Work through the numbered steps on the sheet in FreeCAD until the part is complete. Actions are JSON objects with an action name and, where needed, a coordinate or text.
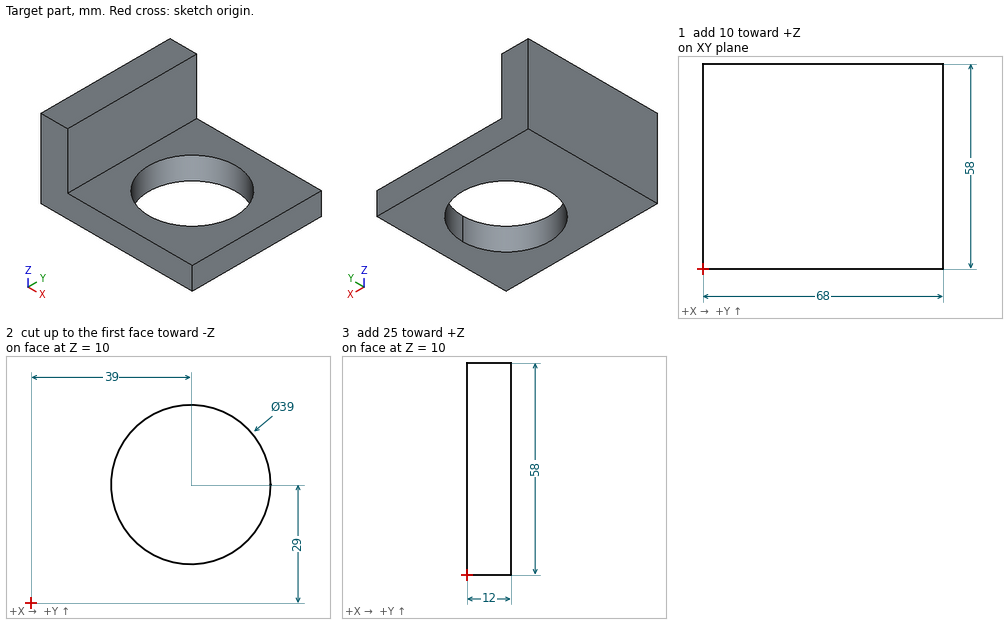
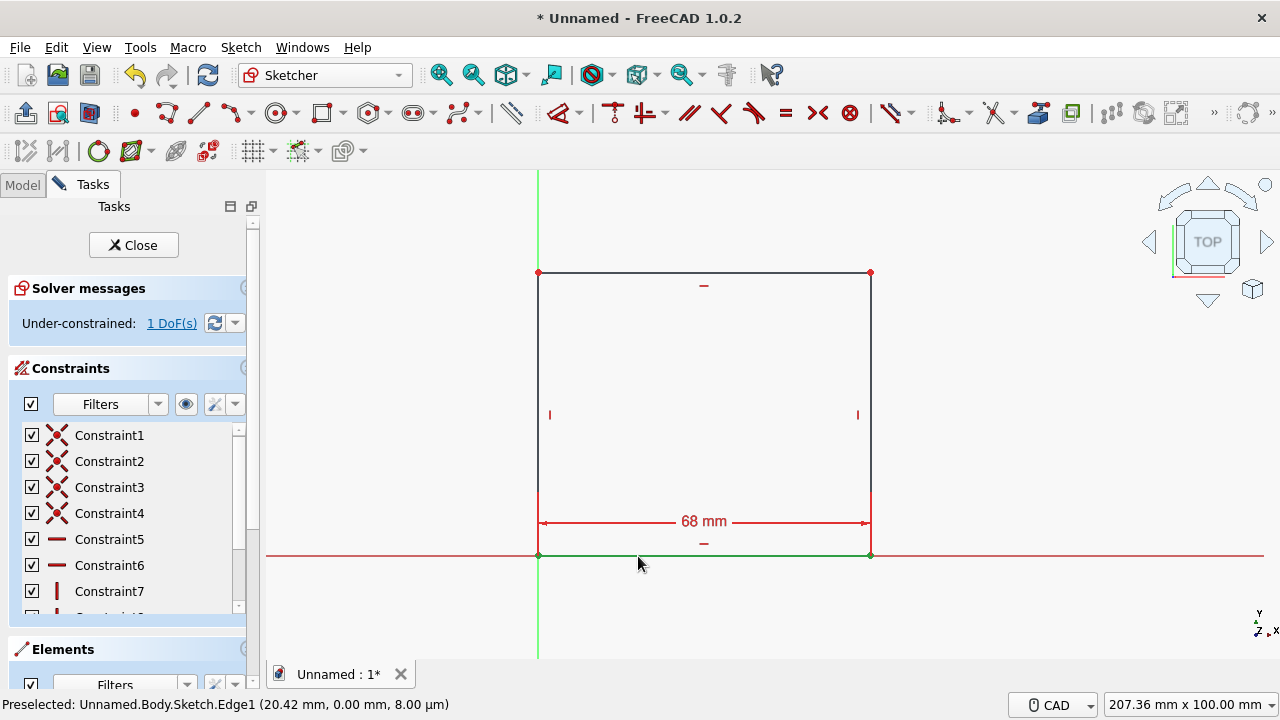
{"action": "left_click", "coordinate": [871, 471]}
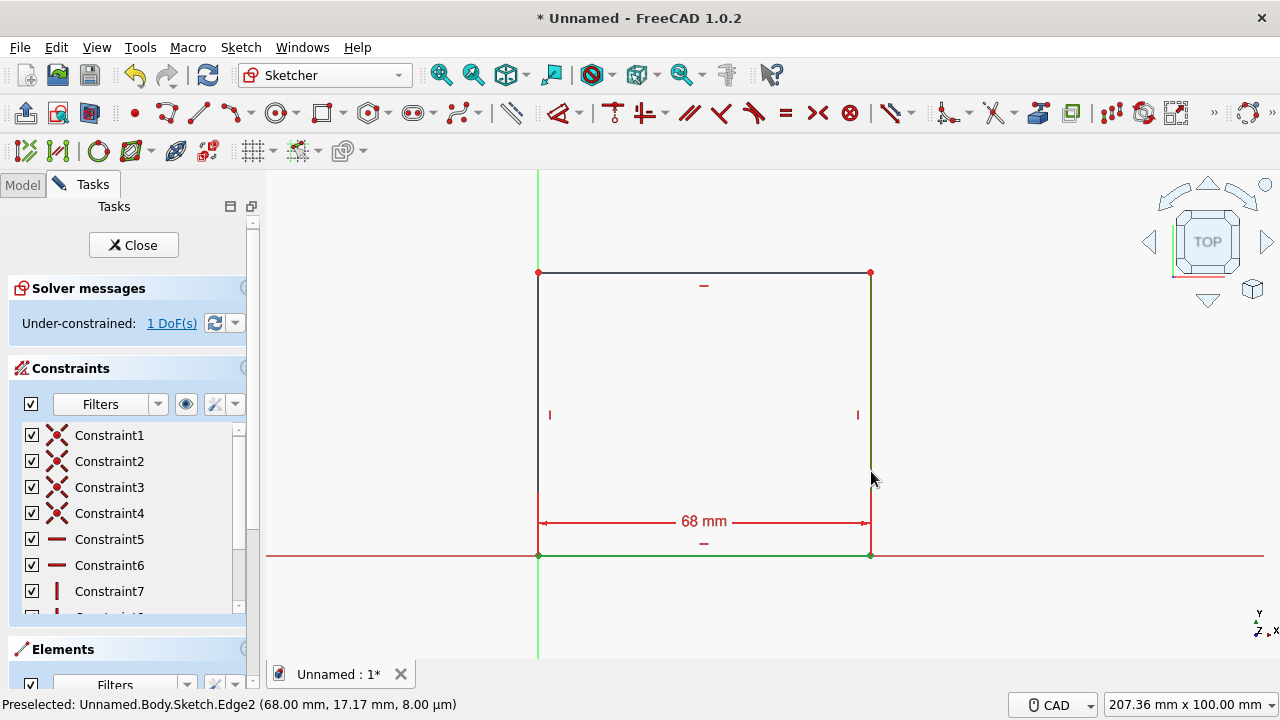
{"action": "left_click", "coordinate": [582, 114]}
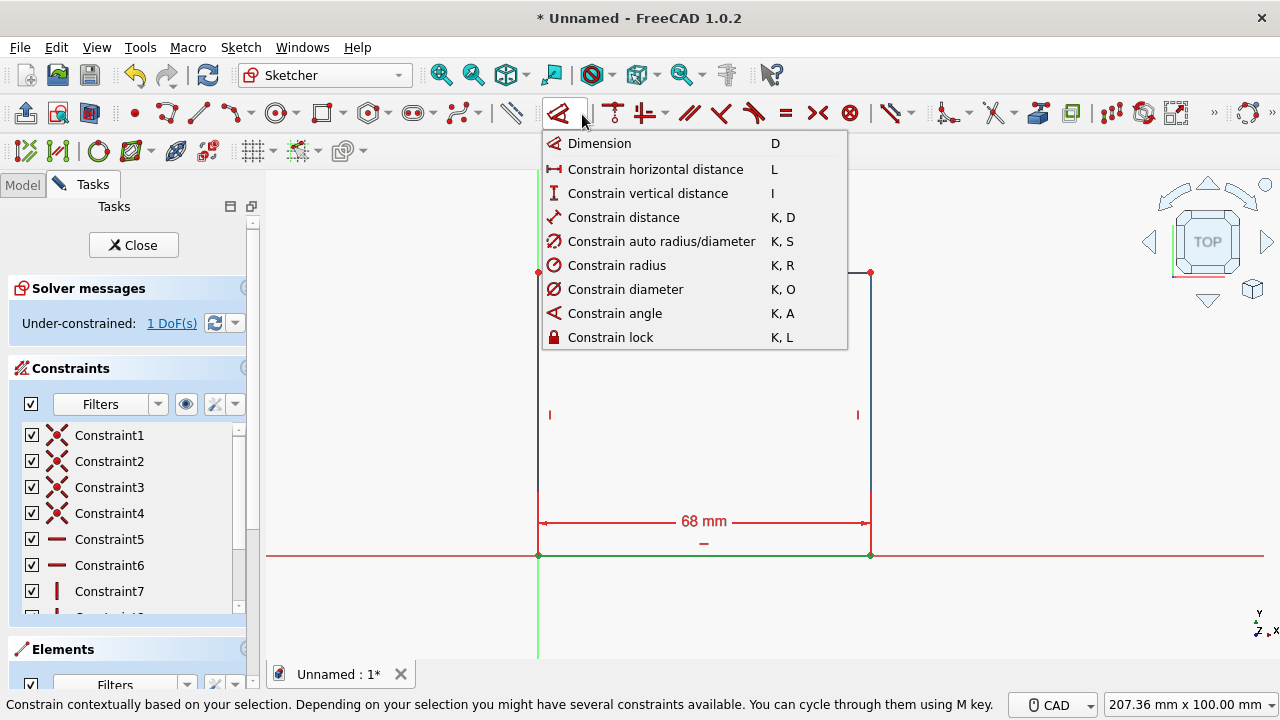
{"action": "left_click", "coordinate": [695, 193]}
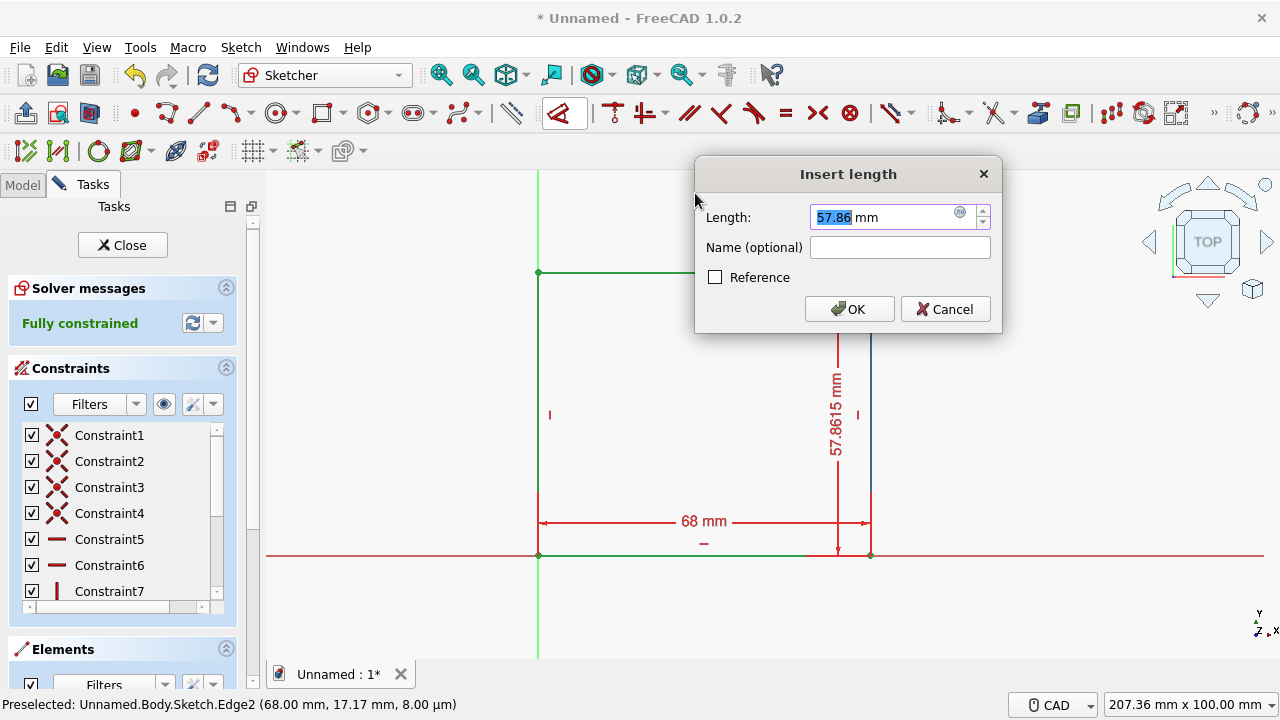
{"action": "type", "text": "58"}
{"action": "key", "text": "Return"}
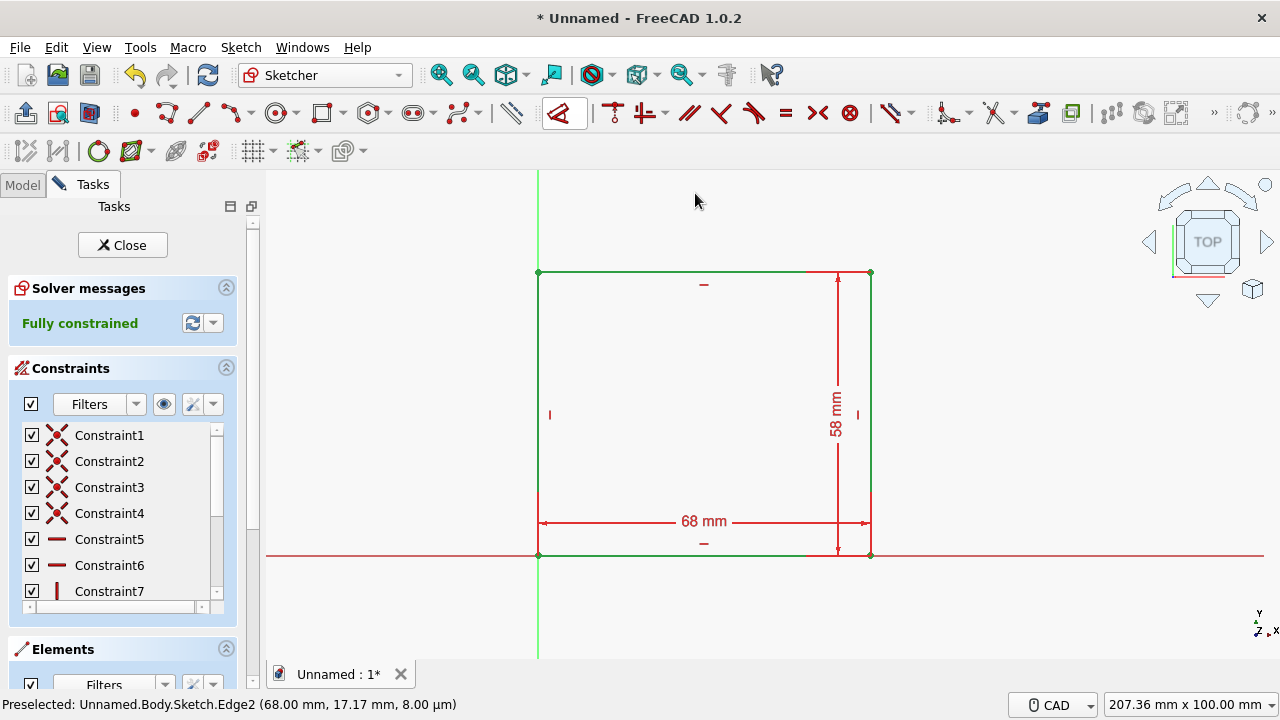
{"action": "left_click", "coordinate": [123, 245]}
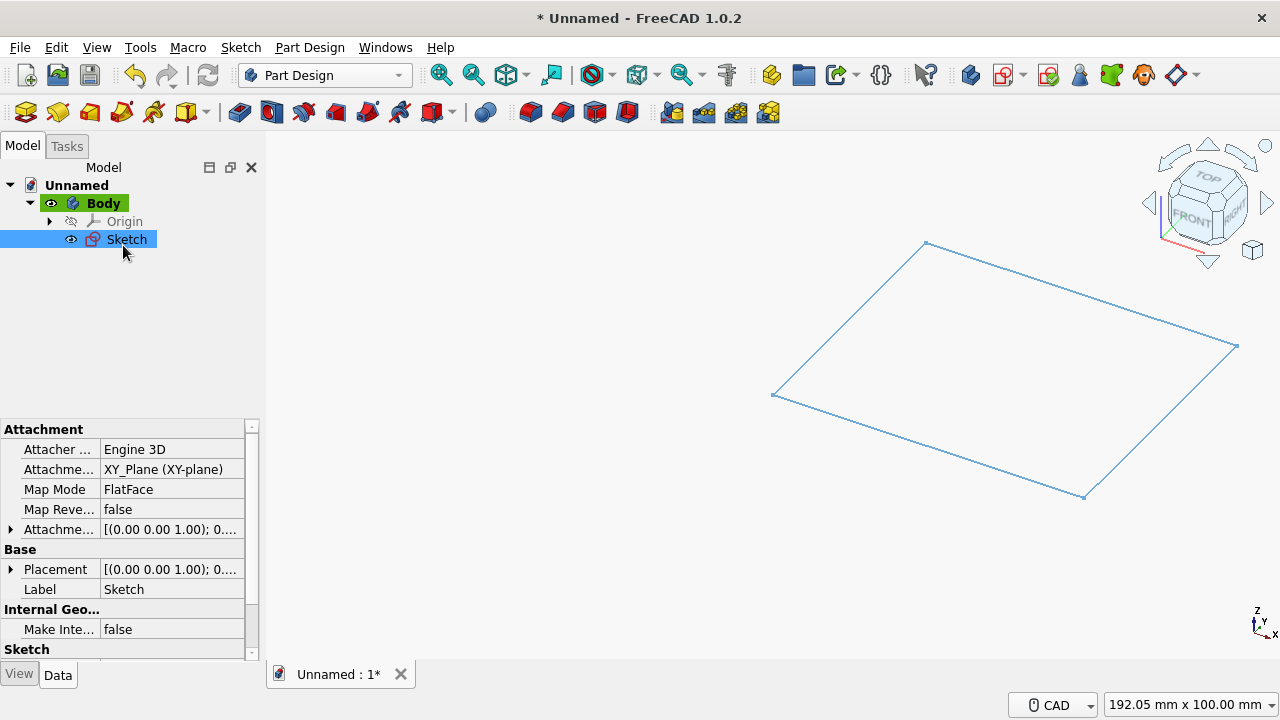
{"action": "left_click", "coordinate": [26, 112]}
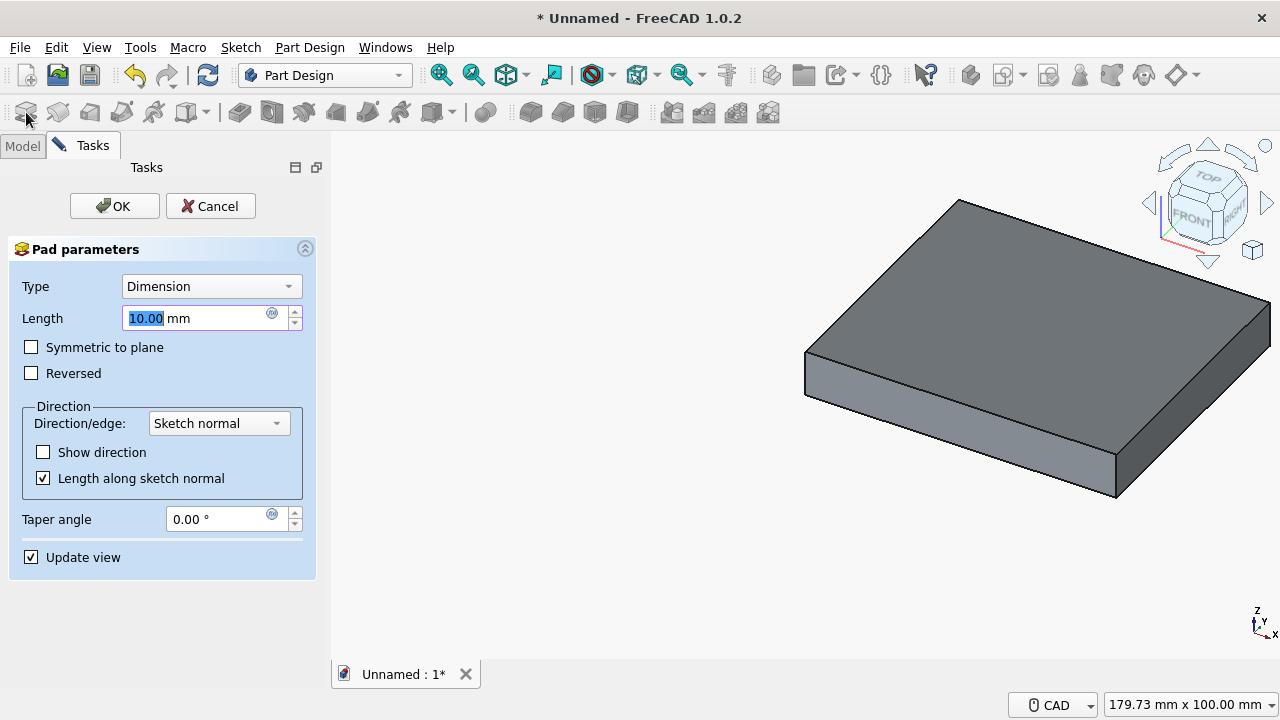
{"action": "type", "text": "10"}
{"action": "key", "text": "Tab"}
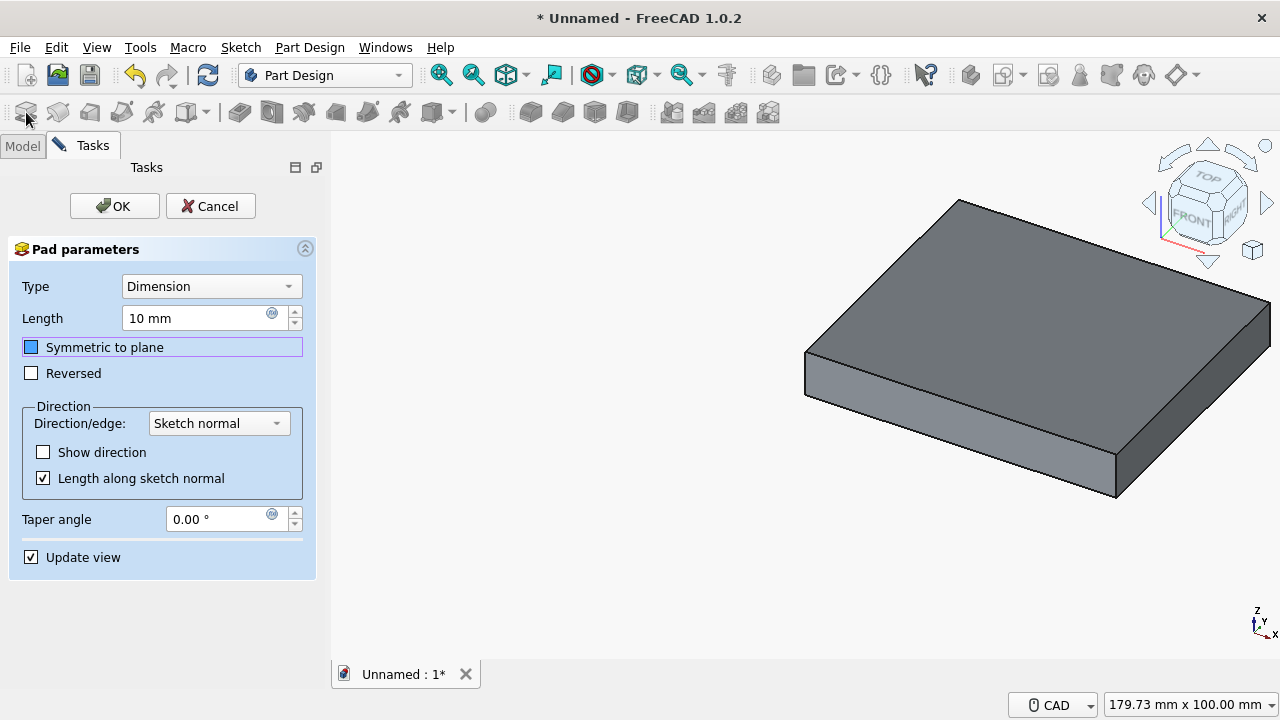
{"action": "left_click", "coordinate": [115, 206]}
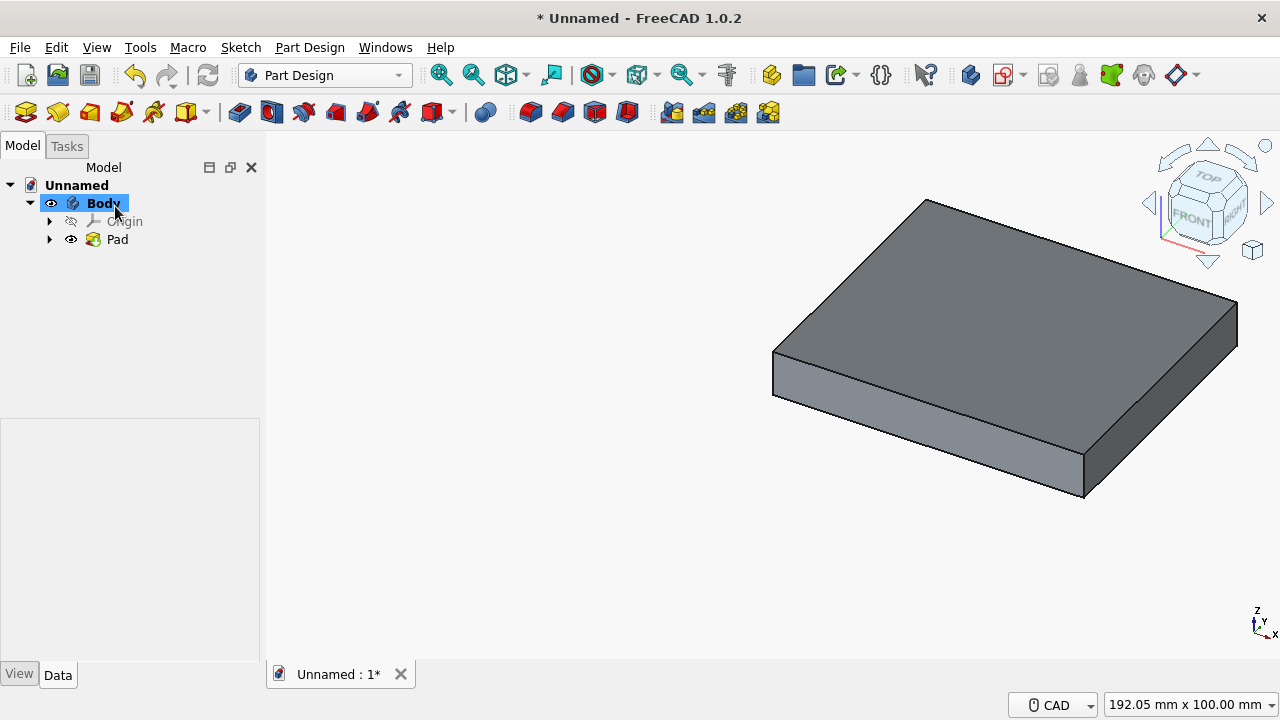
{"action": "left_click", "coordinate": [1005, 326]}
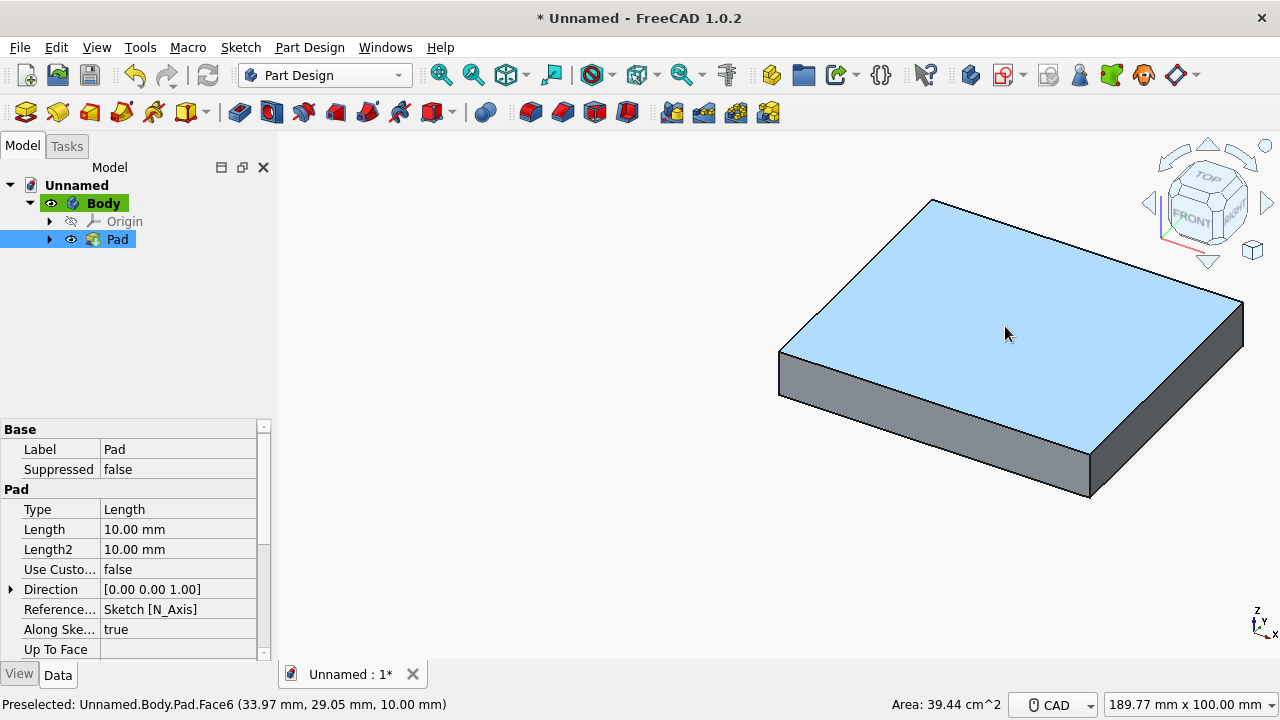
{"action": "left_click", "coordinate": [1004, 76]}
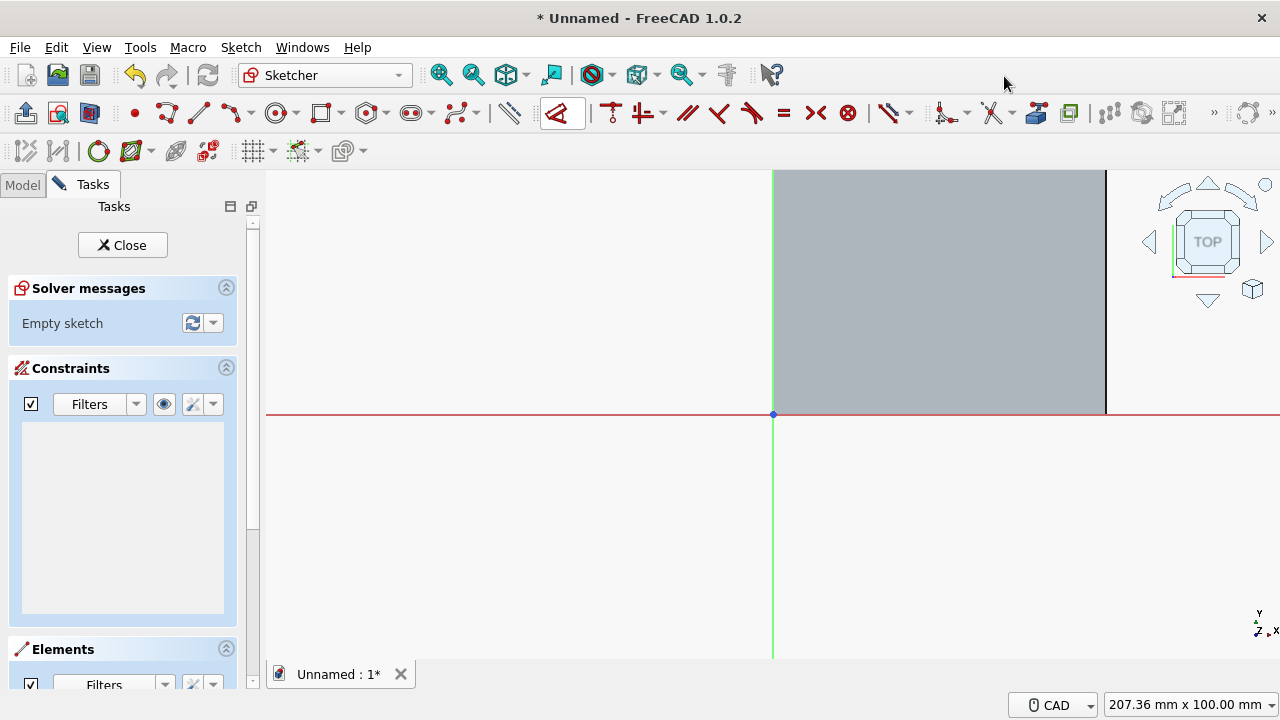
{"action": "scroll", "coordinate": [294, 631], "scroll_direction": "down", "scroll_amount": 1}